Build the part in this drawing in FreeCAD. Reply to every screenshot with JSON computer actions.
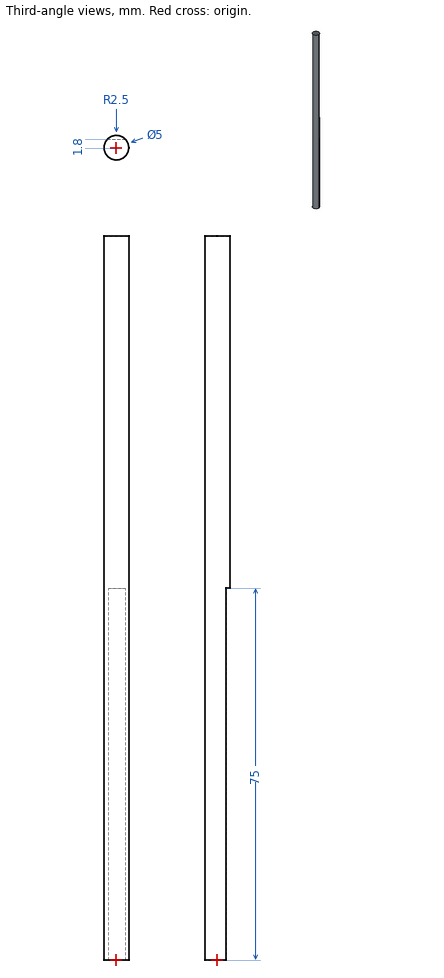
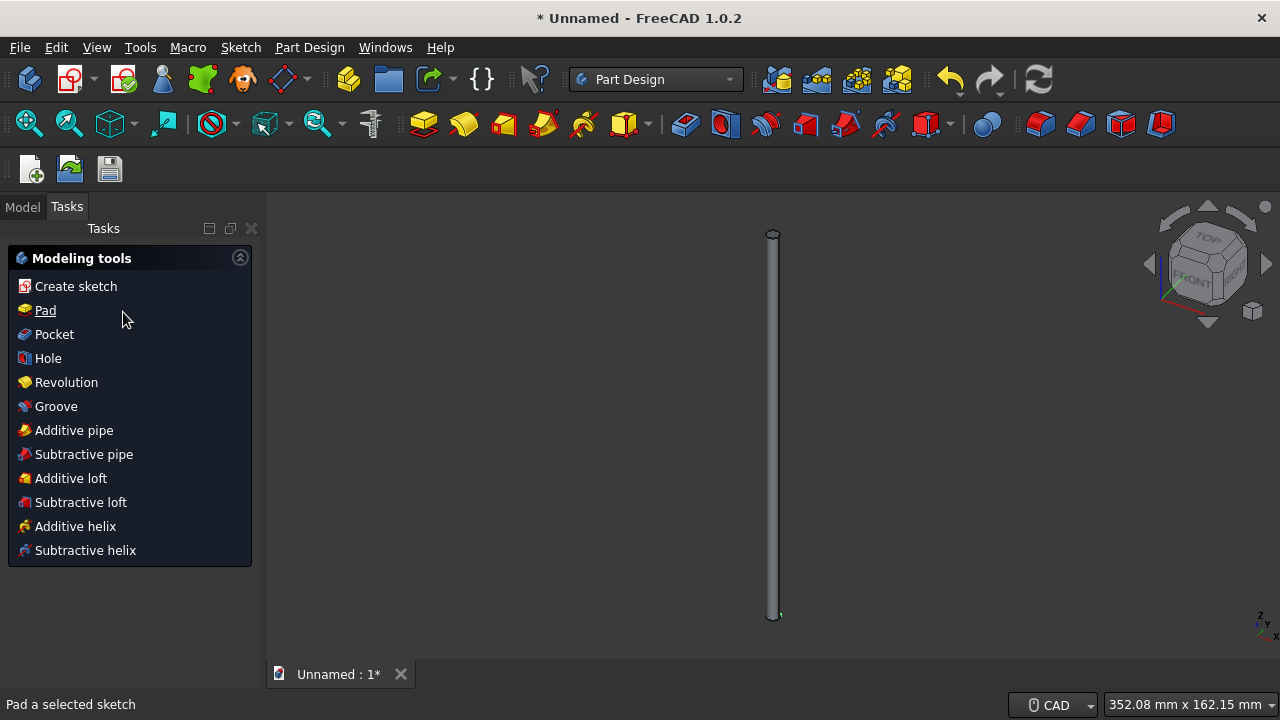
{"action": "left_click", "coordinate": [686, 124]}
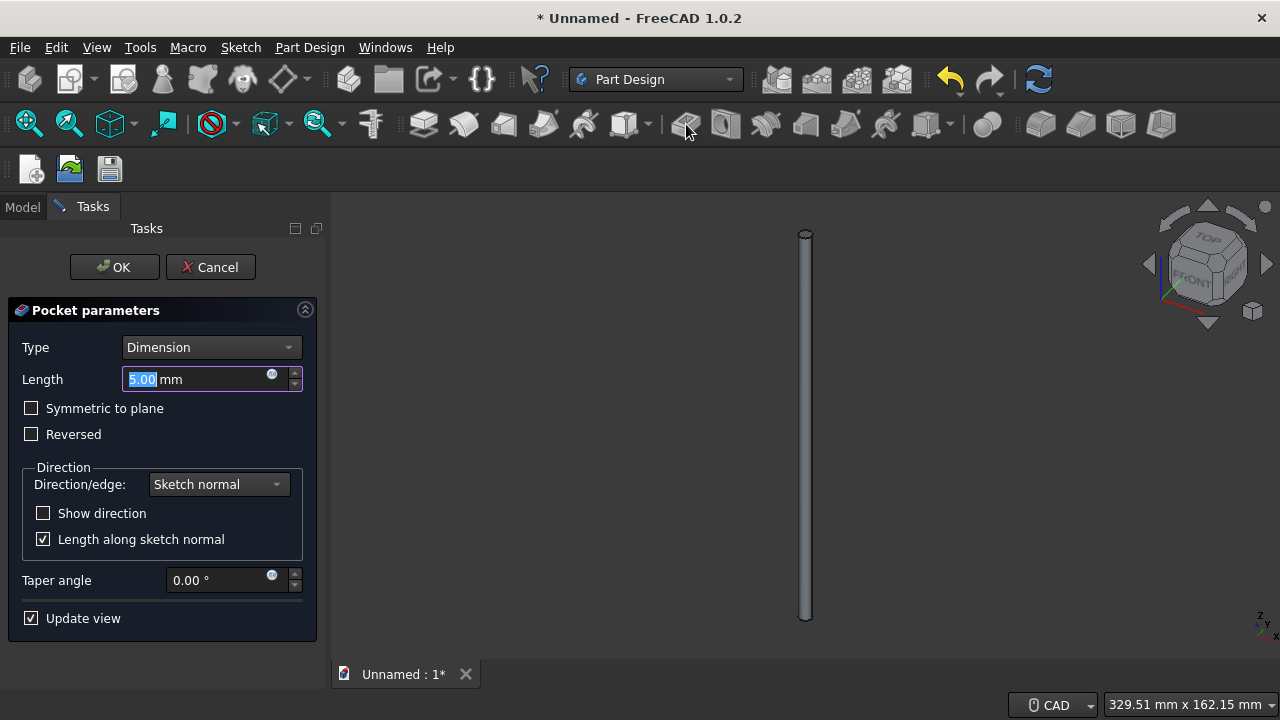
{"action": "type", "text": "75"}
{"action": "key", "text": "Tab"}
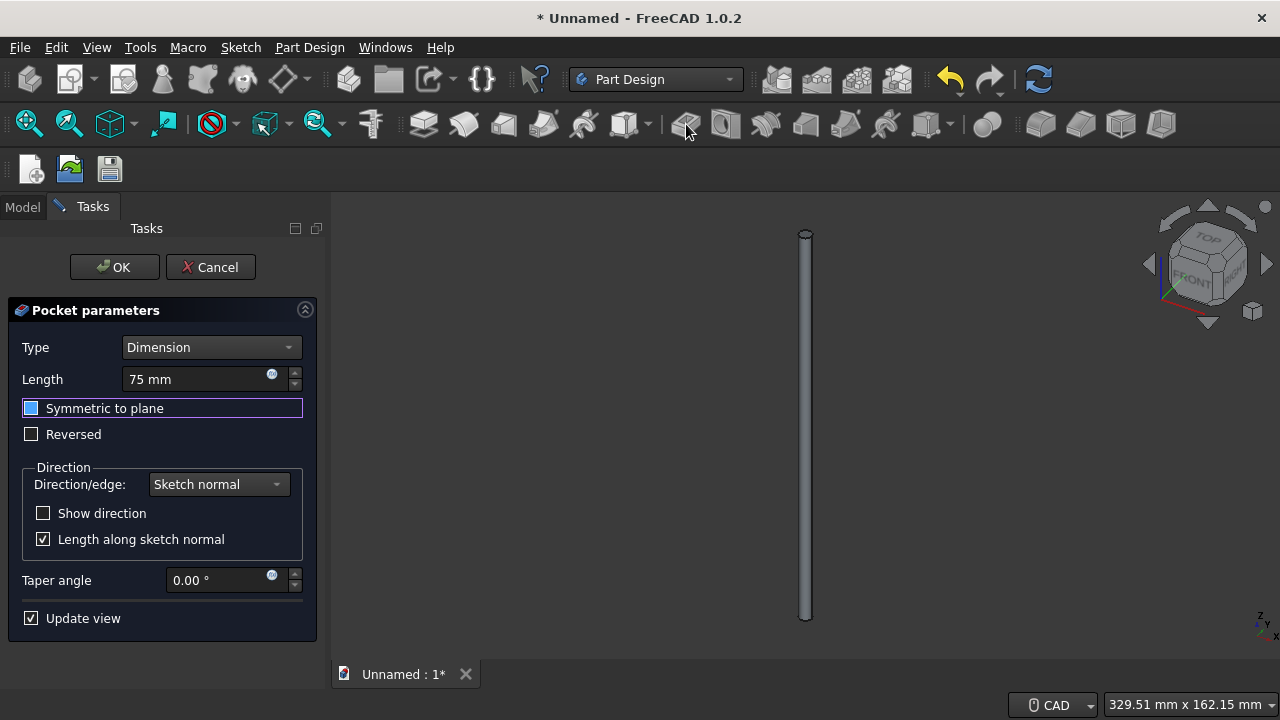
{"action": "left_click", "coordinate": [30, 434]}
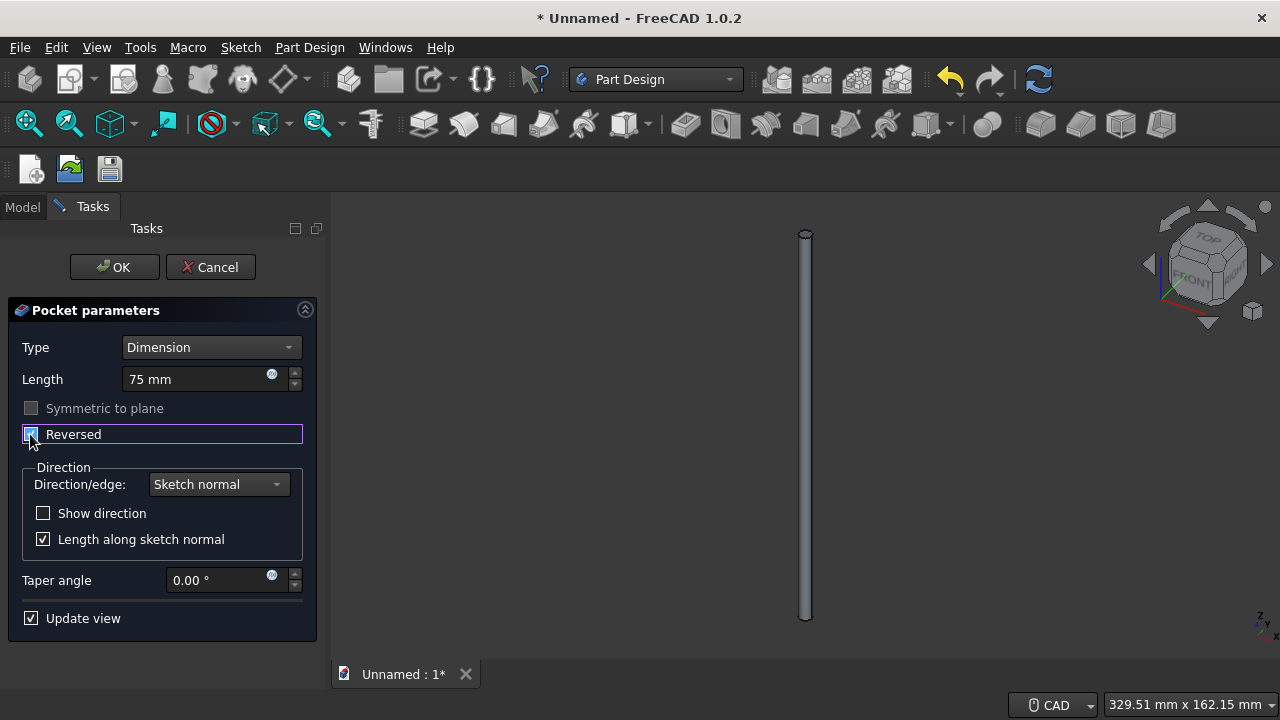
{"action": "left_click", "coordinate": [115, 267]}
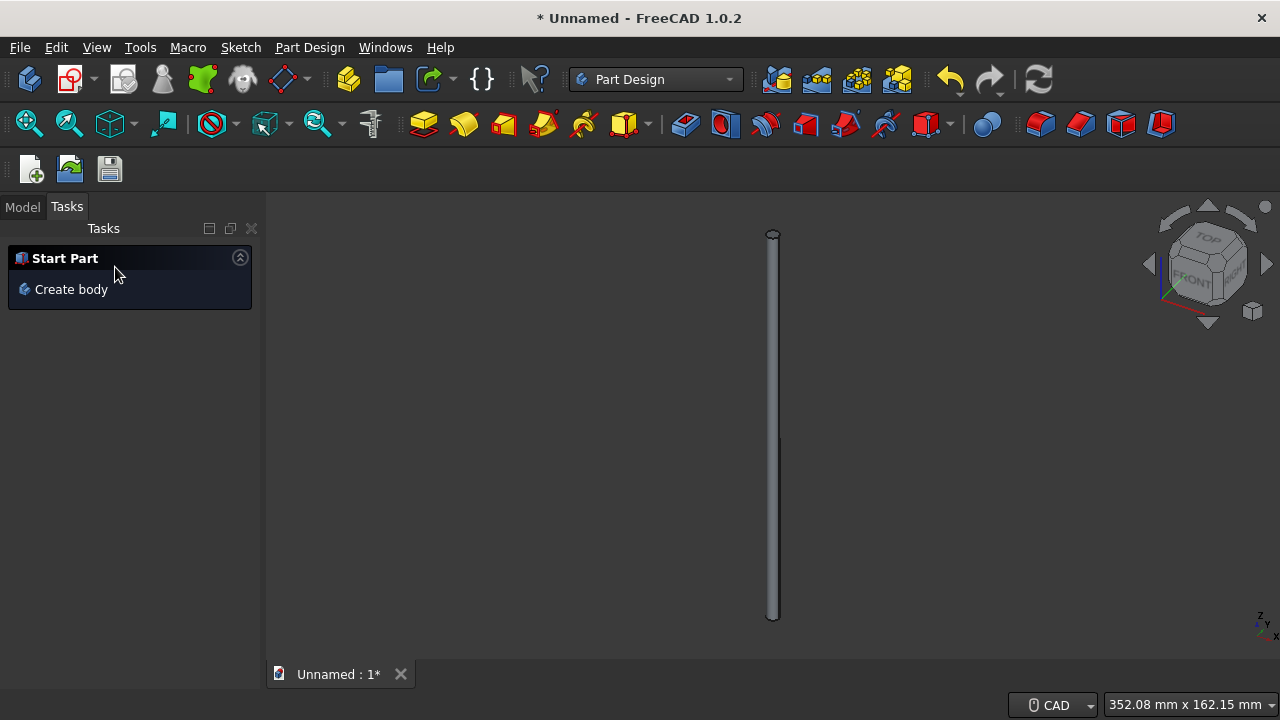
{"action": "left_click", "coordinate": [23, 206]}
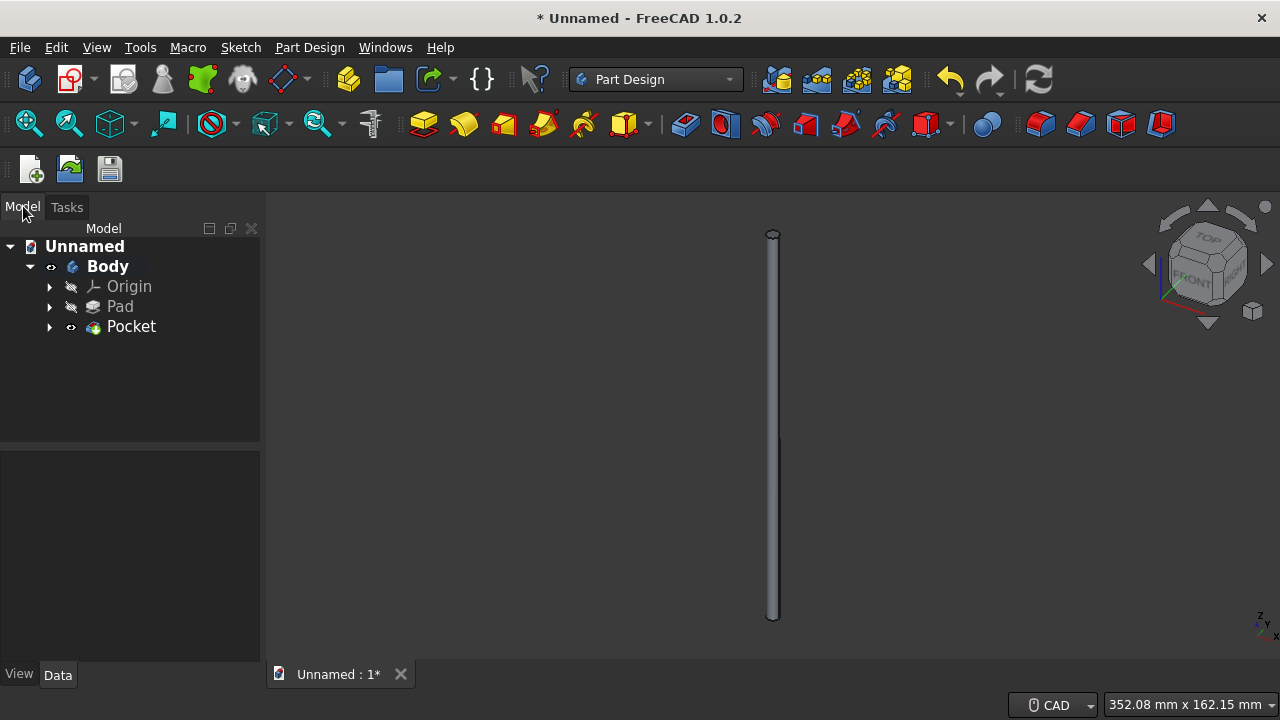
{"action": "left_click", "coordinate": [50, 287]}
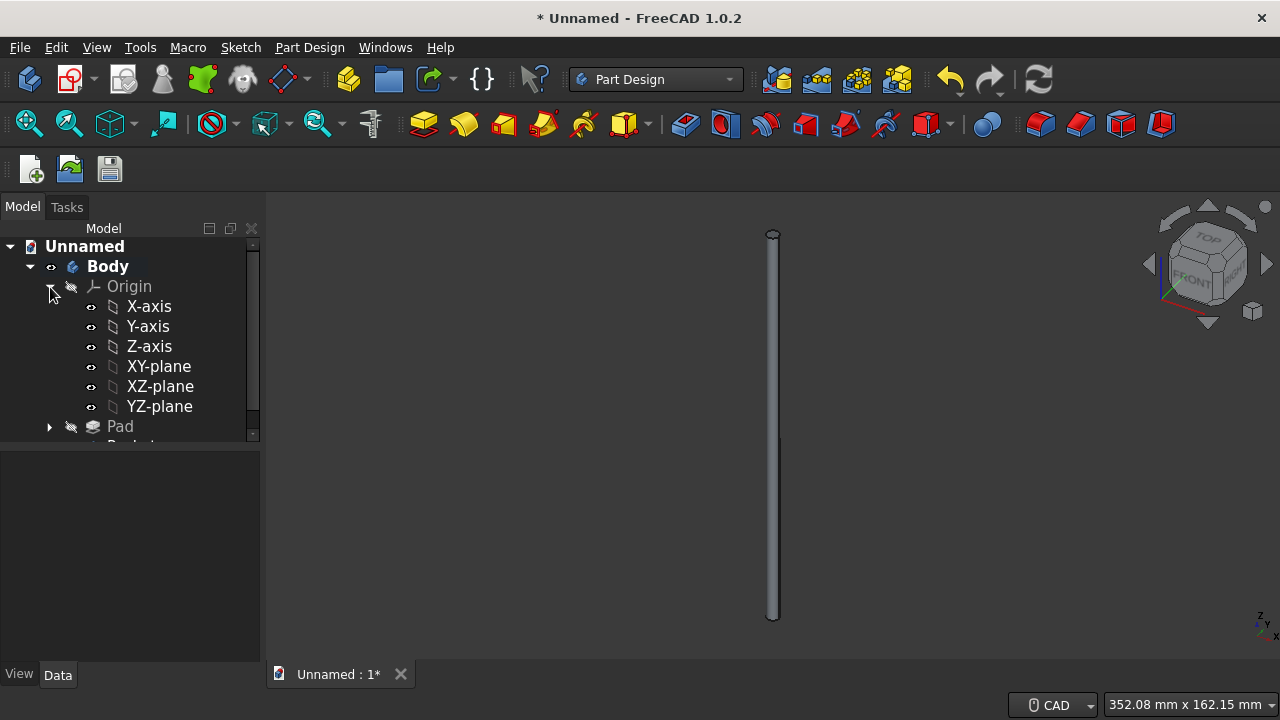
{"action": "left_click", "coordinate": [136, 367]}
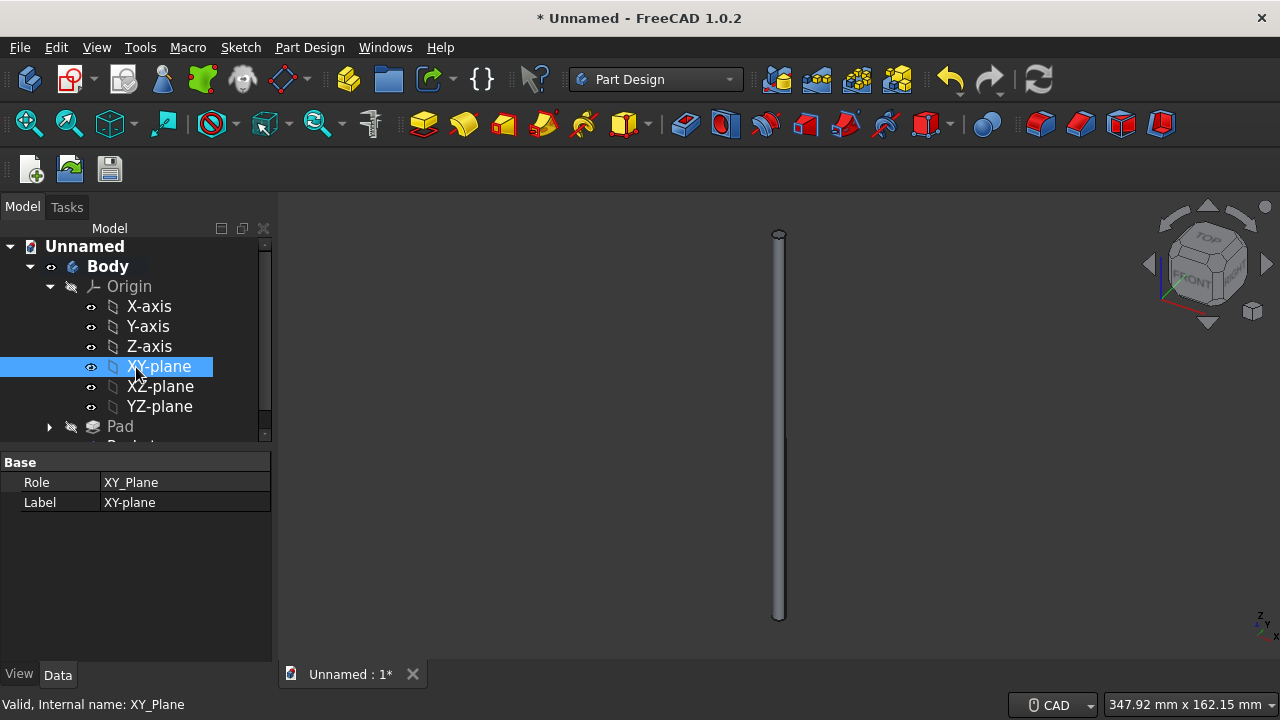
{"action": "left_click", "coordinate": [284, 80]}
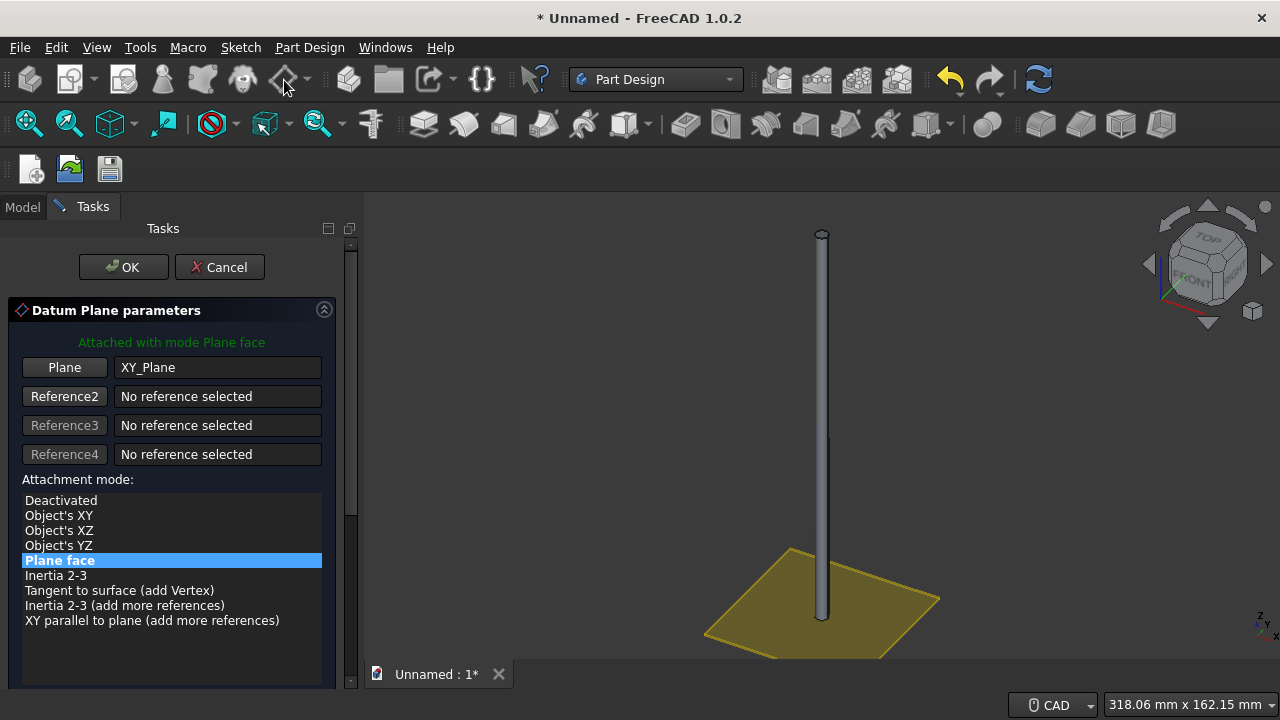
{"action": "scroll", "coordinate": [351, 463], "scroll_direction": "down", "scroll_amount": 3}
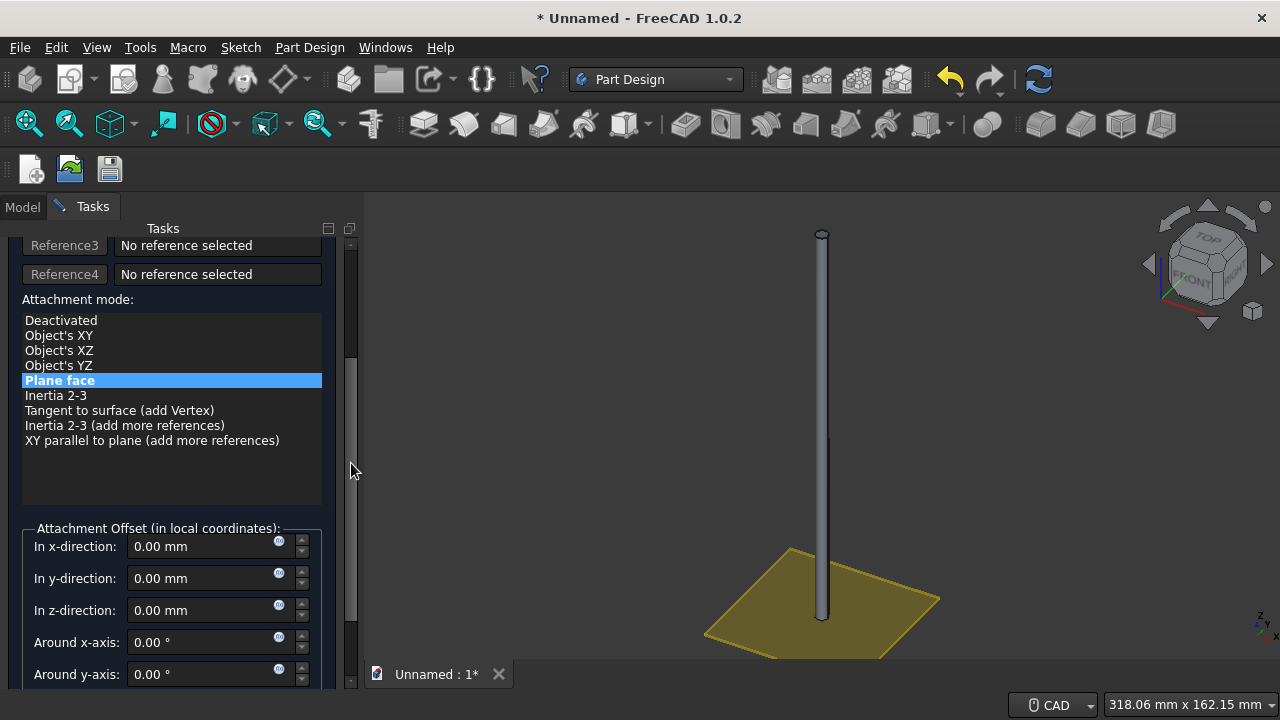
{"action": "triple_click", "coordinate": [210, 610]}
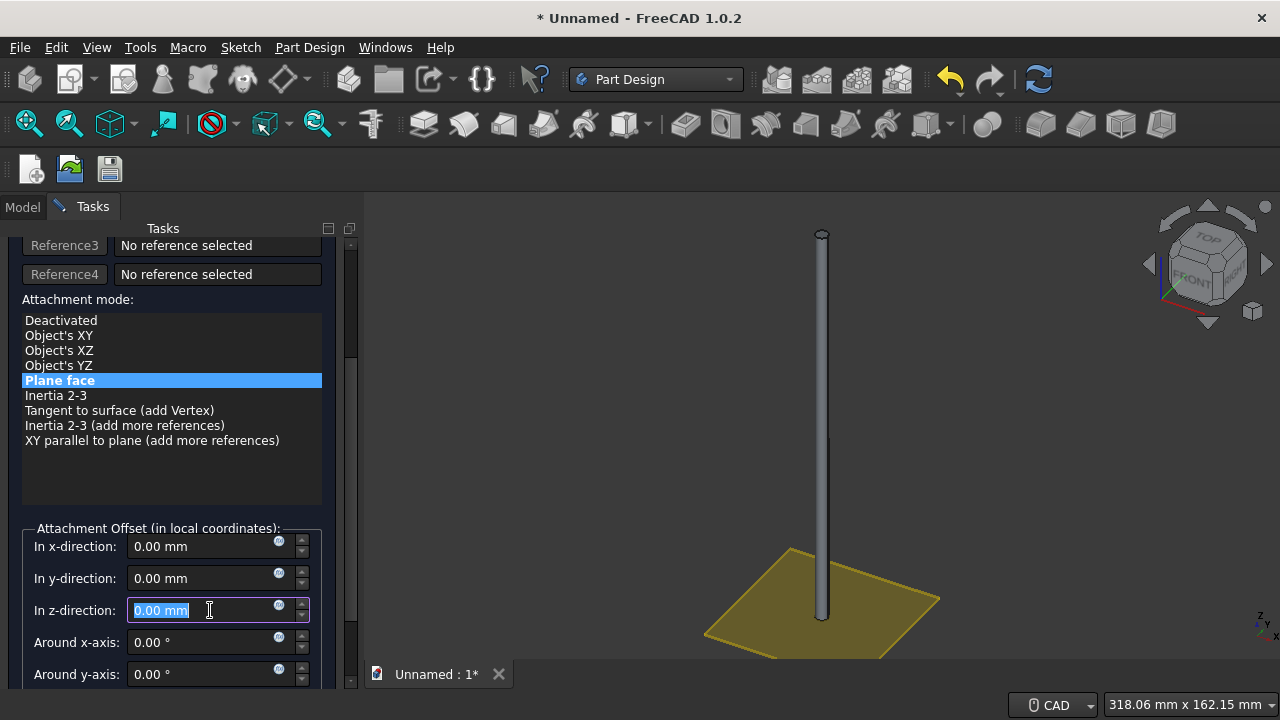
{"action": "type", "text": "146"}
{"action": "key", "text": "Tab"}